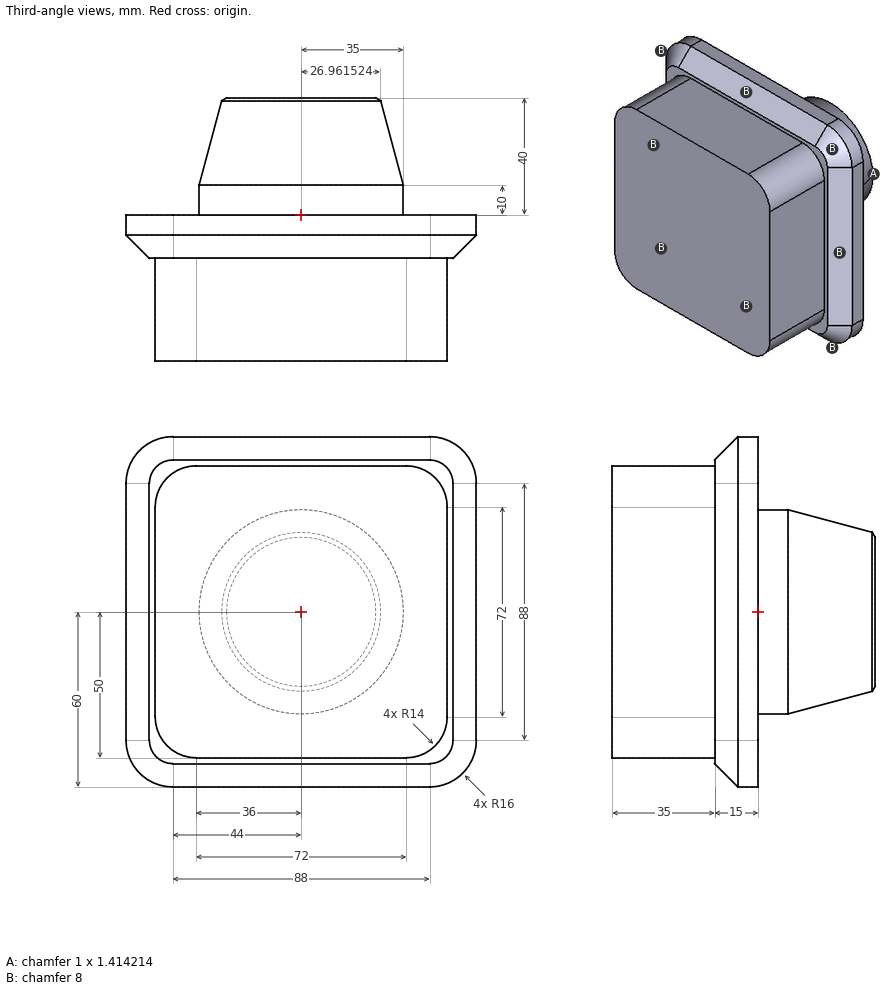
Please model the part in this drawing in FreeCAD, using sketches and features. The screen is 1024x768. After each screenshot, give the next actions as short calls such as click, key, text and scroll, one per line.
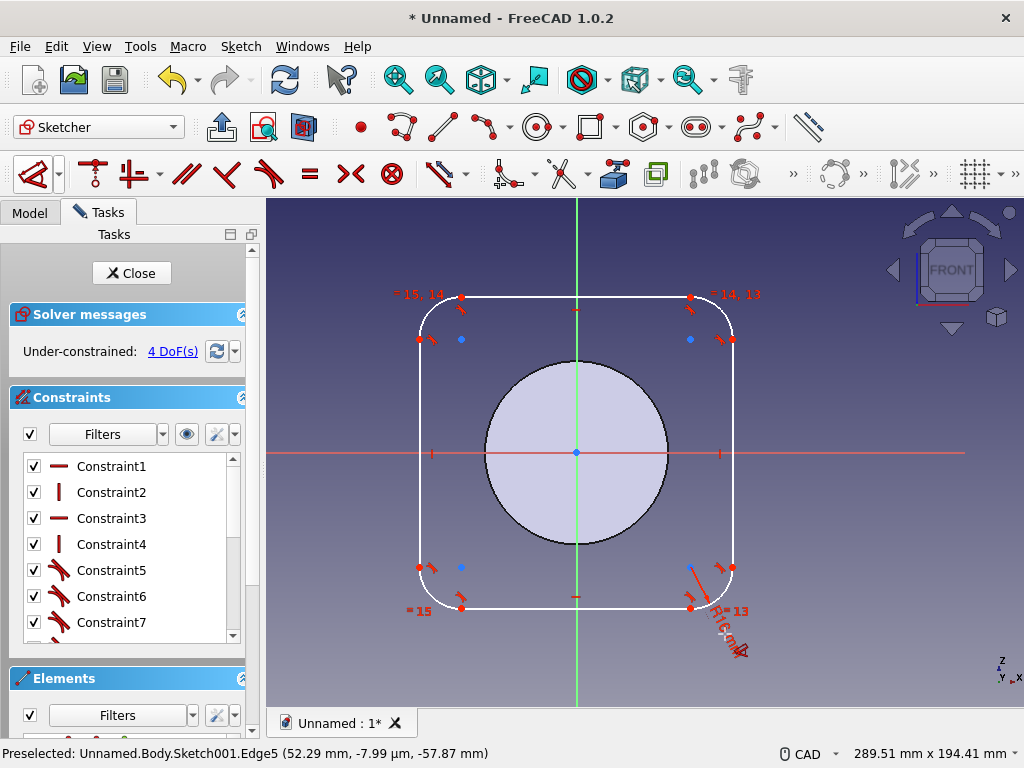
click(530, 609)
click(523, 643)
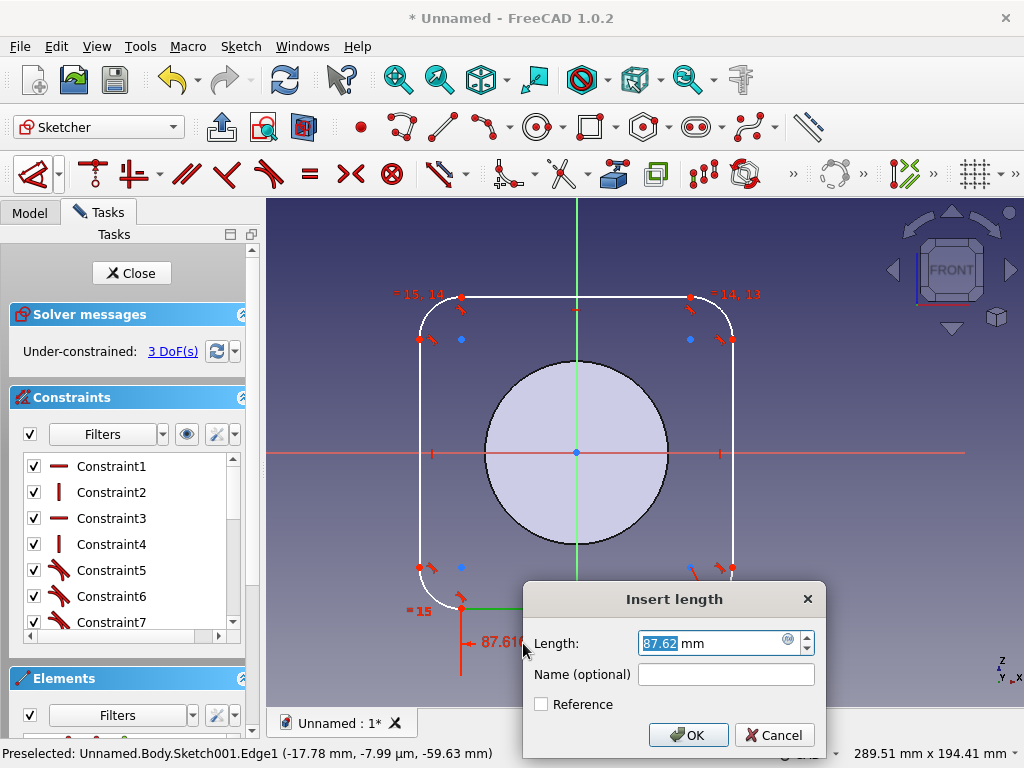
text(88)
key(Return)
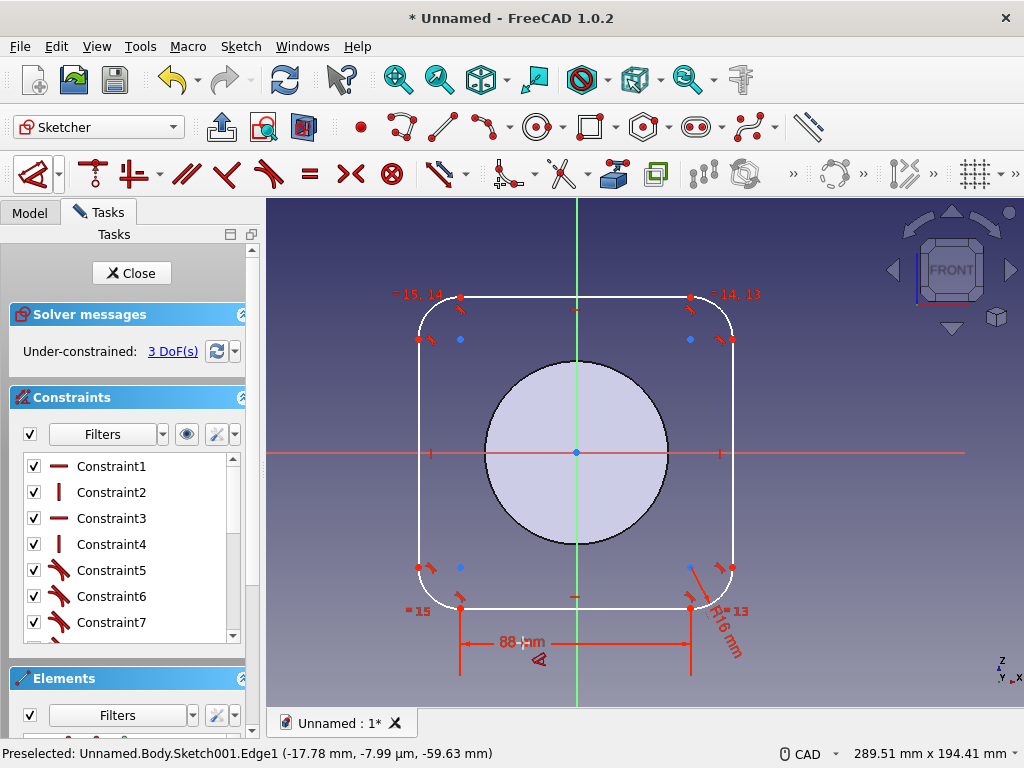
click(733, 499)
click(767, 401)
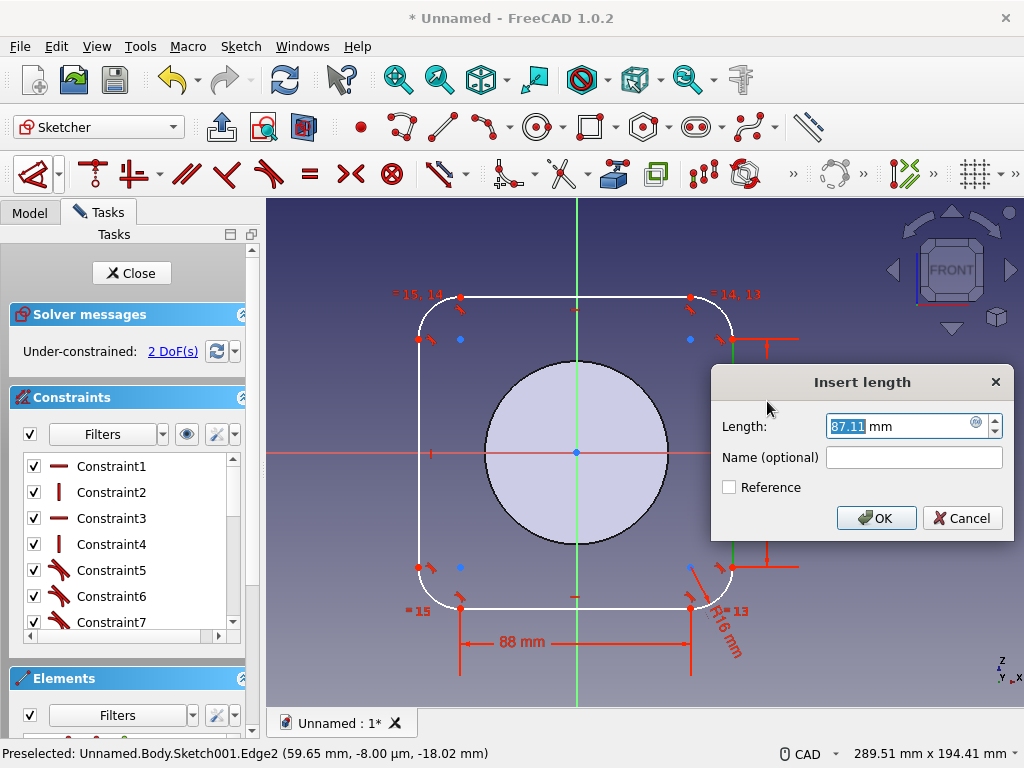
text(88)
key(Return)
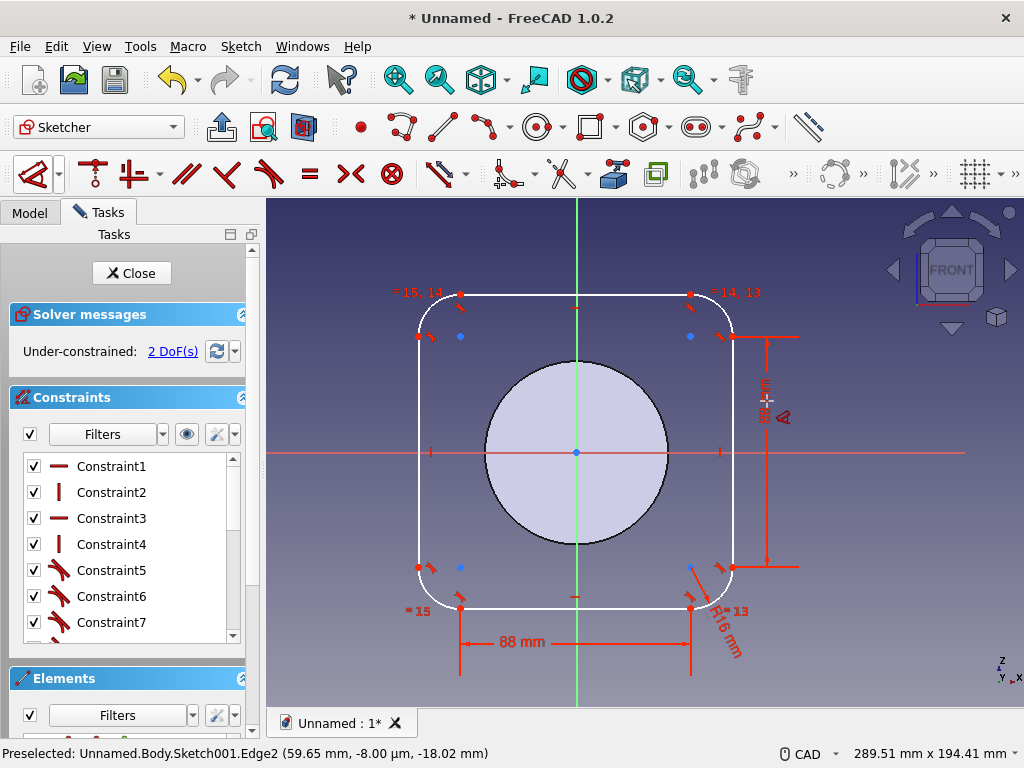
click(460, 609)
click(518, 419)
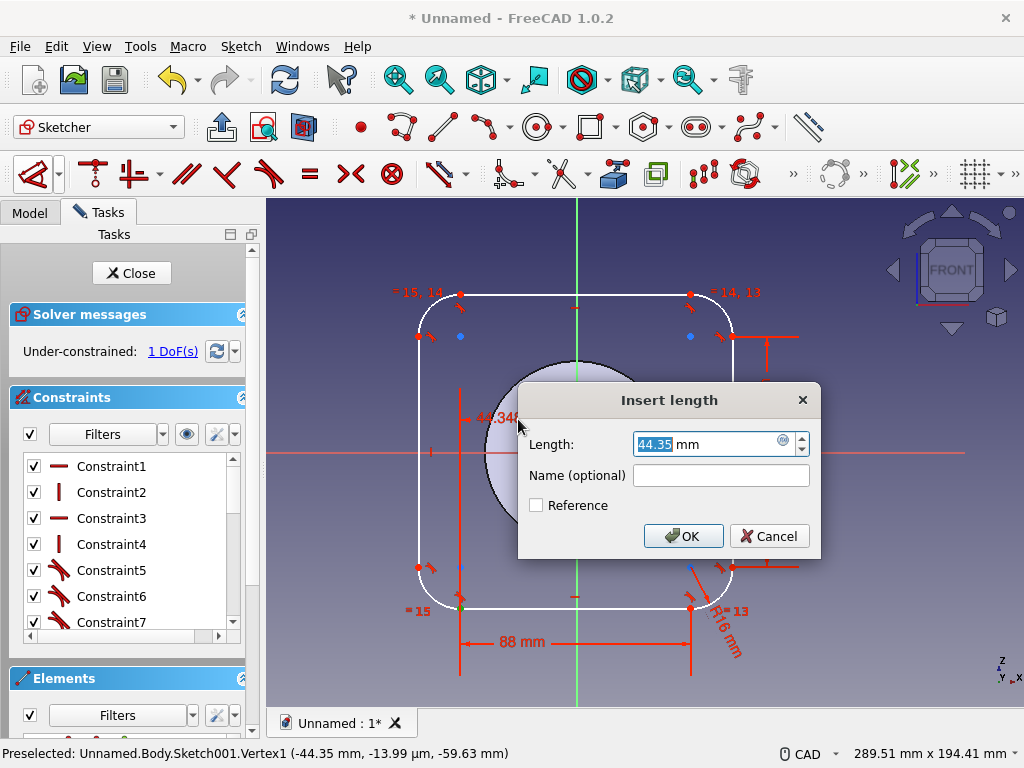
text(44)
key(Return)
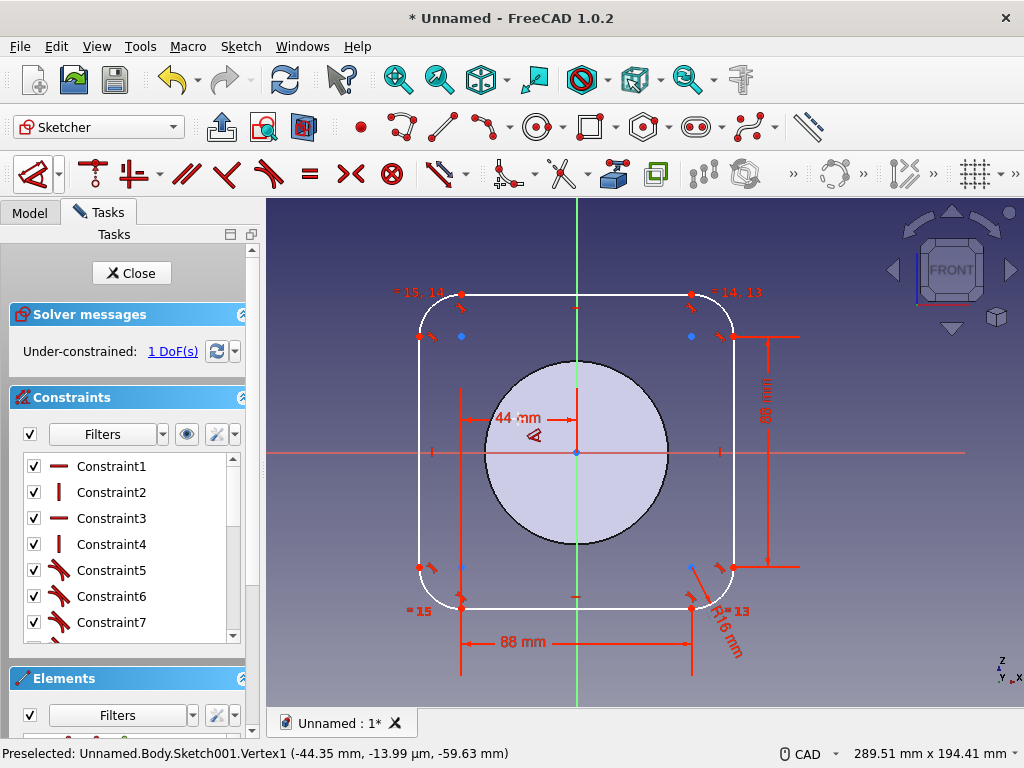
click(461, 609)
click(611, 531)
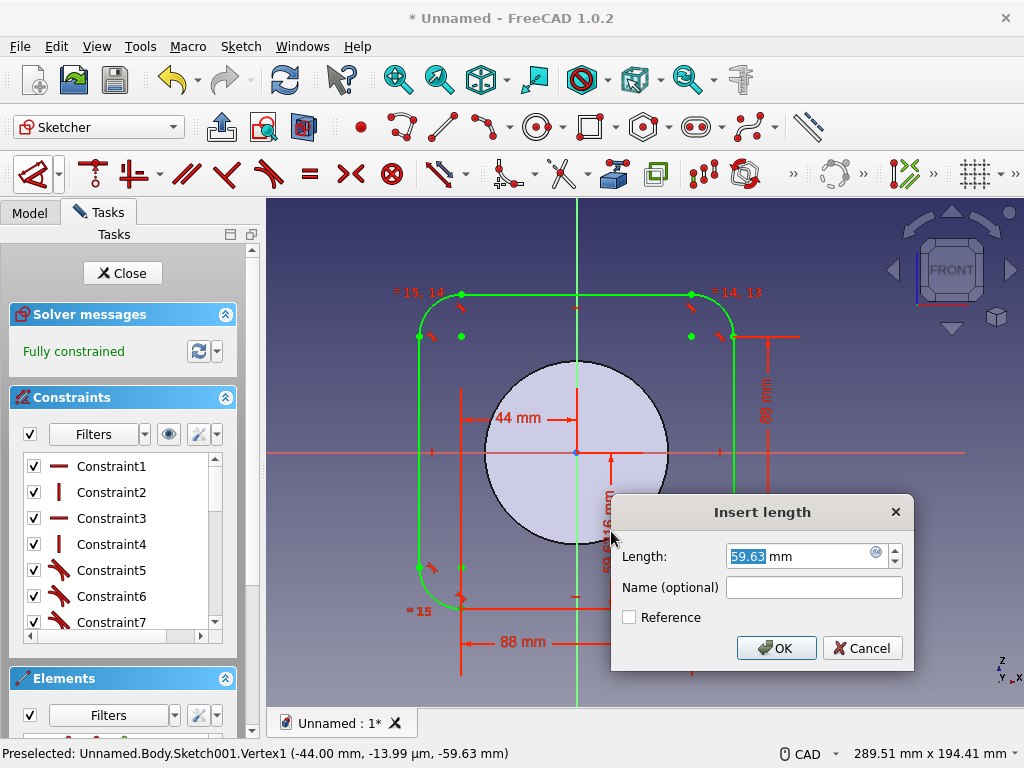
text(60)
key(Return)
key(Escape)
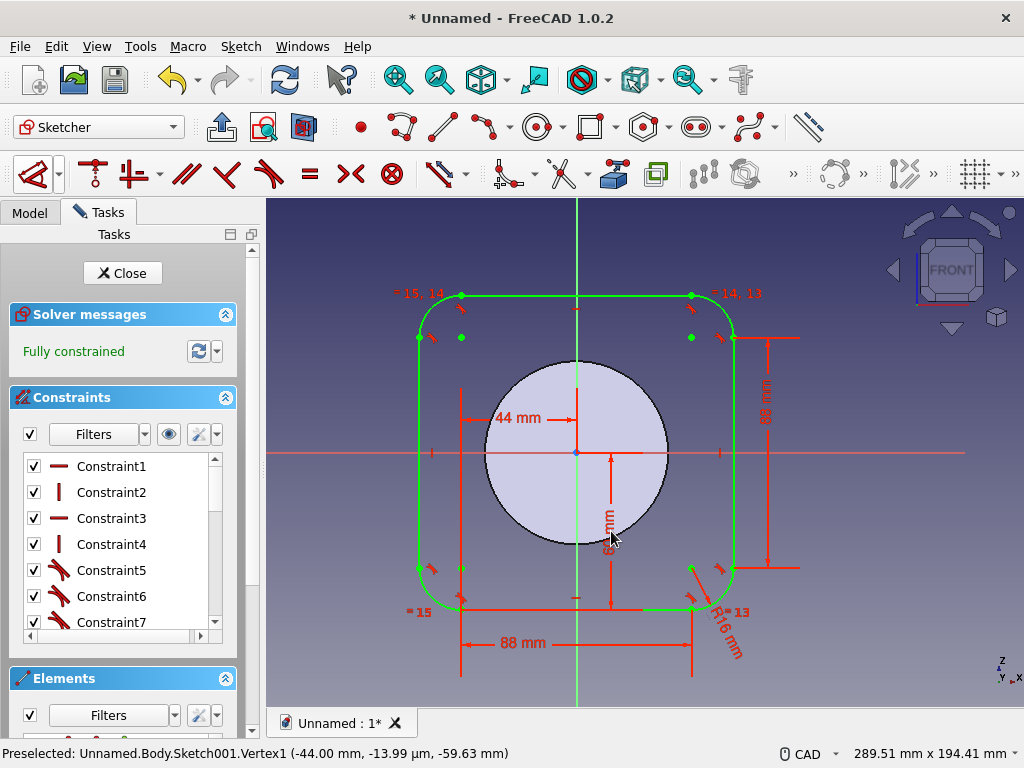
click(123, 273)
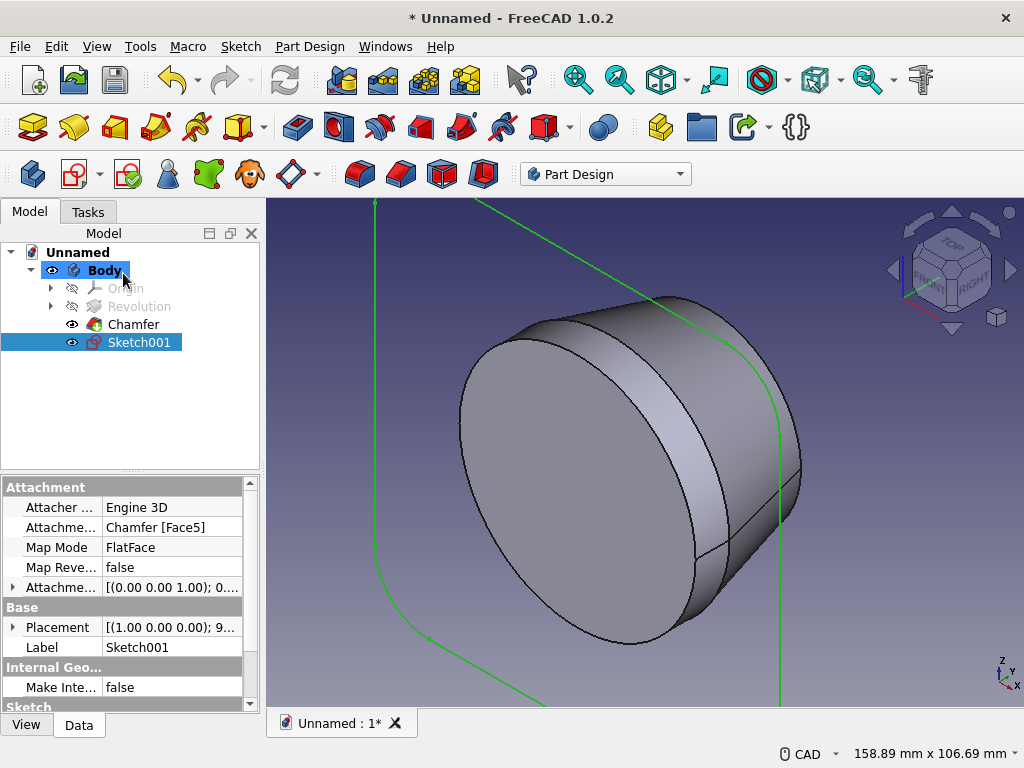
click(33, 128)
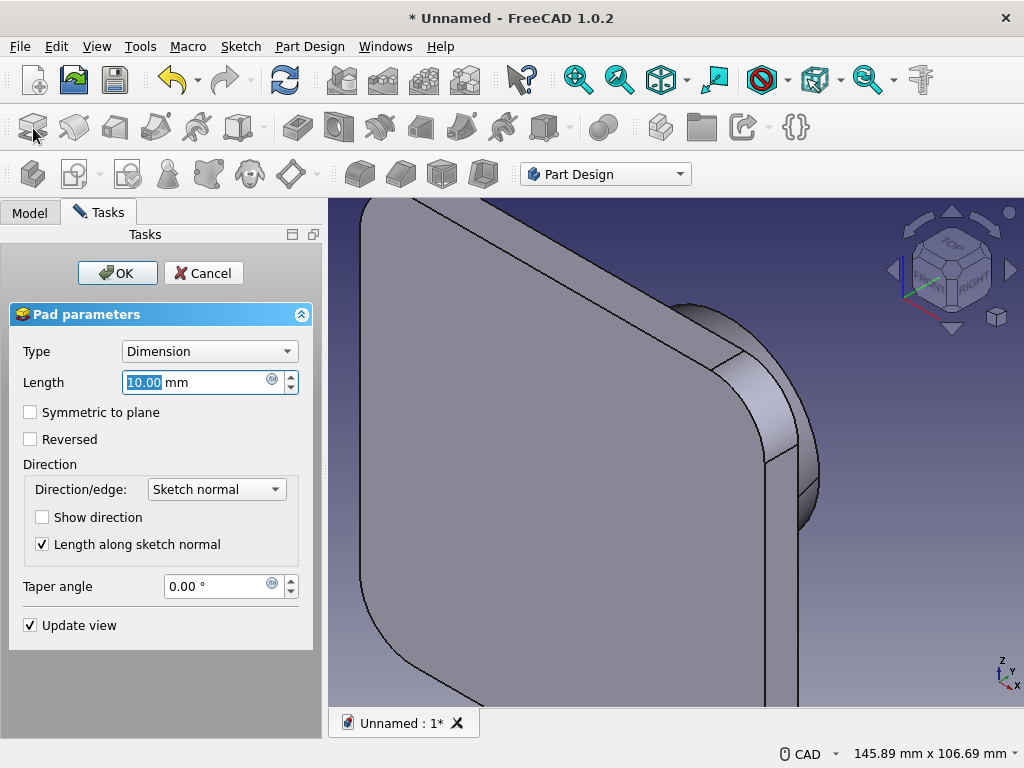
text(15)
key(Tab)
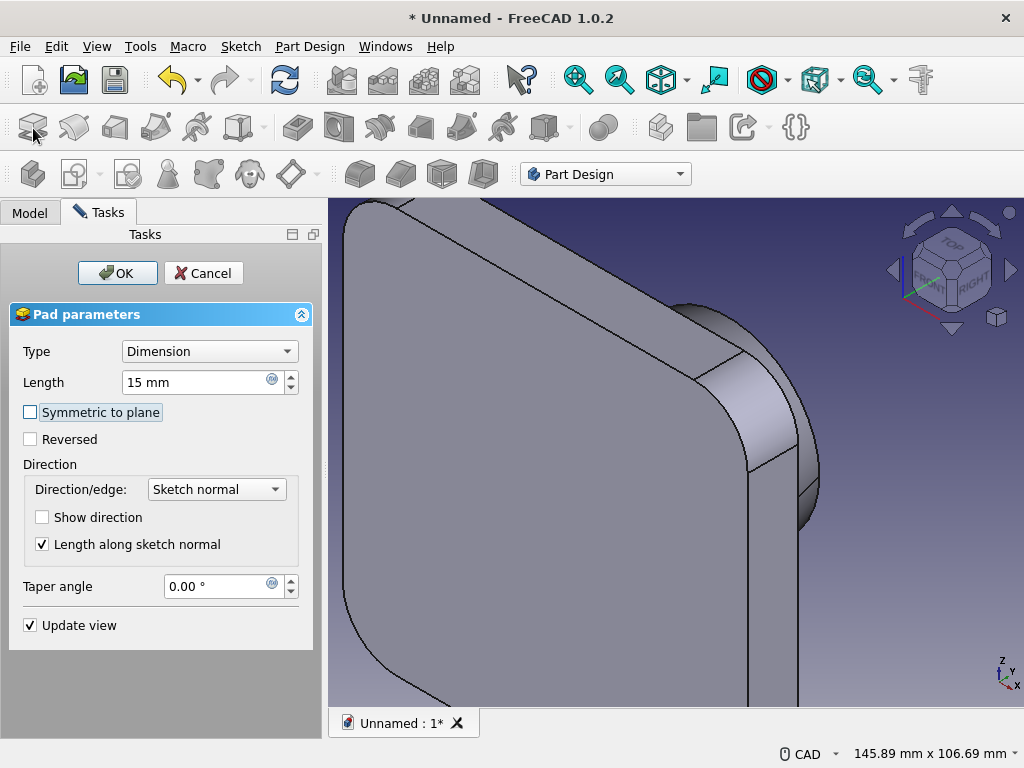
click(118, 273)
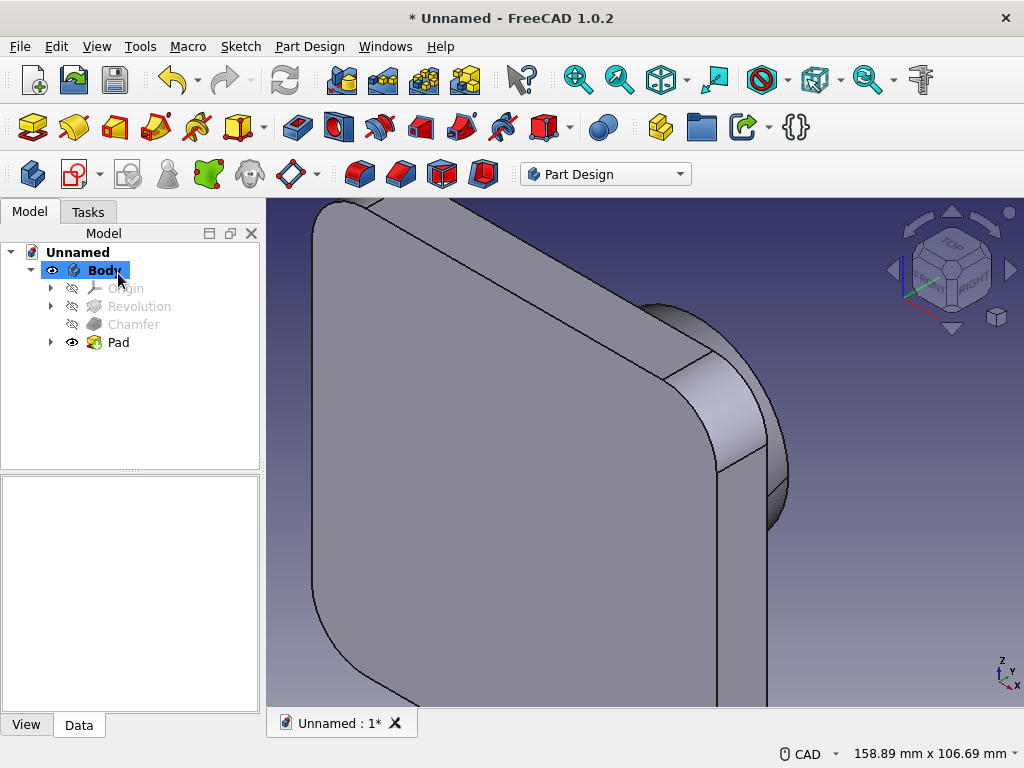
click(579, 80)